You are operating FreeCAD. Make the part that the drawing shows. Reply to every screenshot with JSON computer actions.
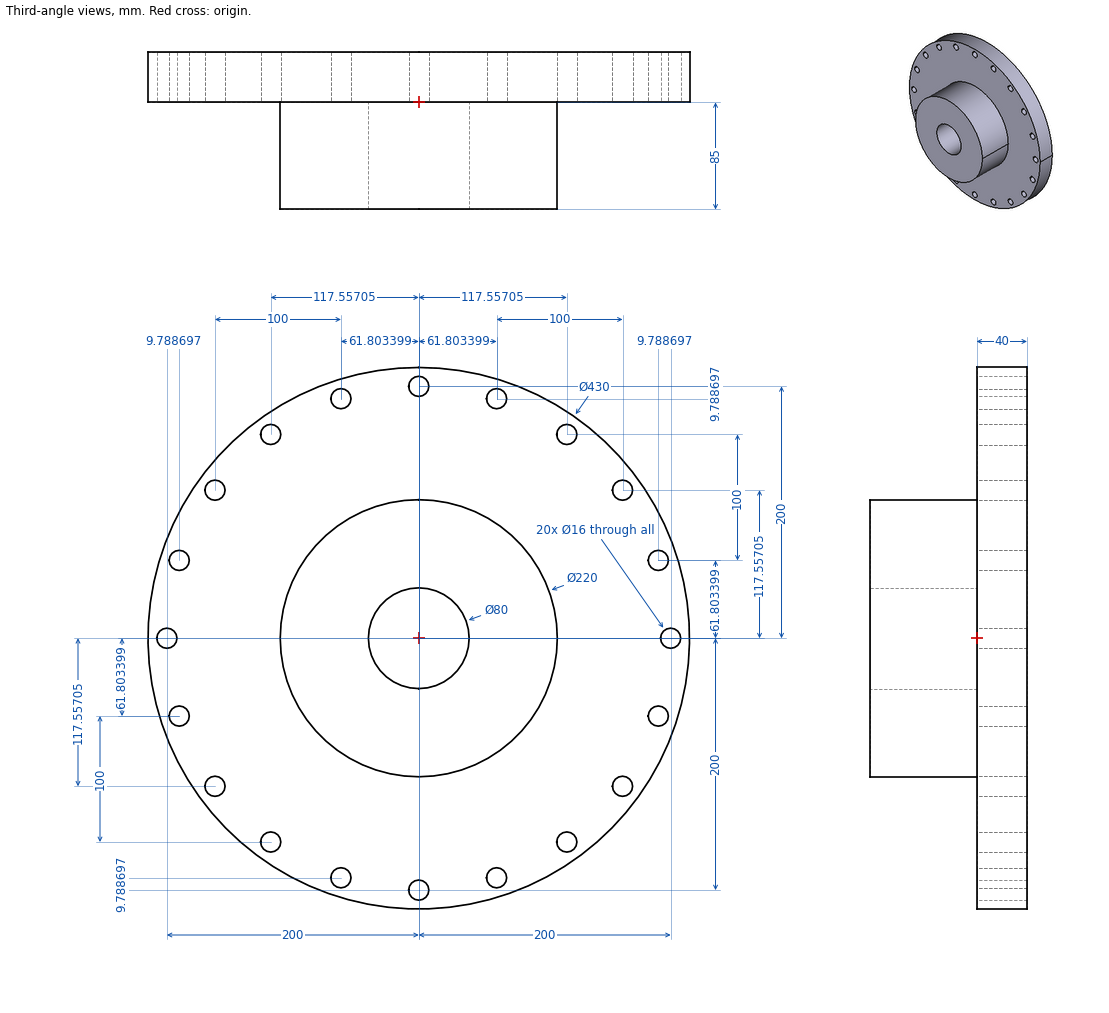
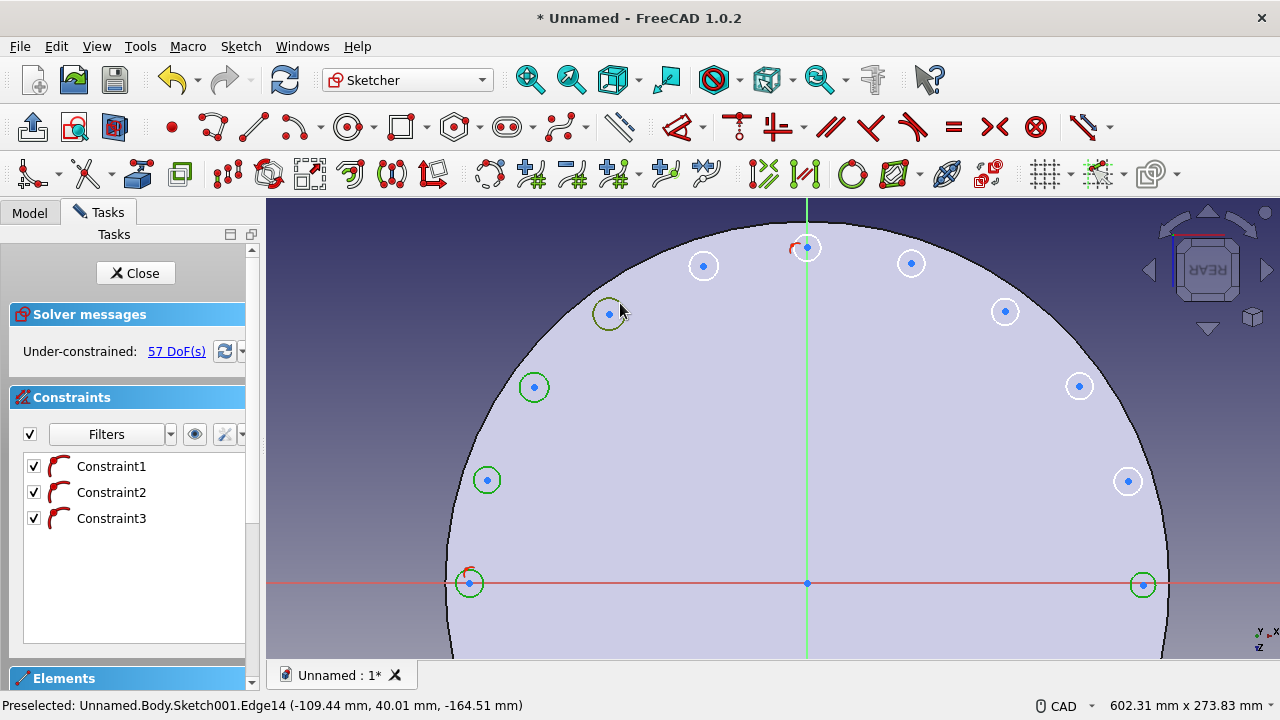
{"action": "left_click", "coordinate": [714, 256]}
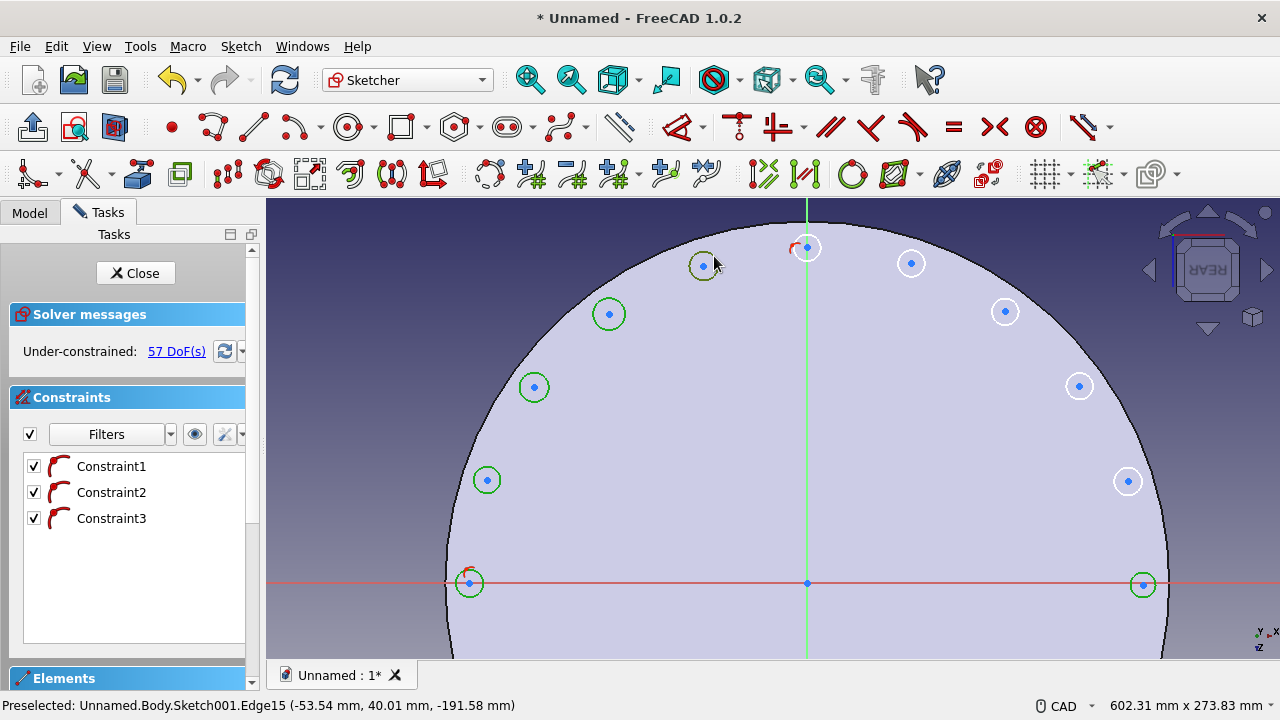
{"action": "scroll", "coordinate": [817, 238], "scroll_direction": "up", "scroll_amount": 2}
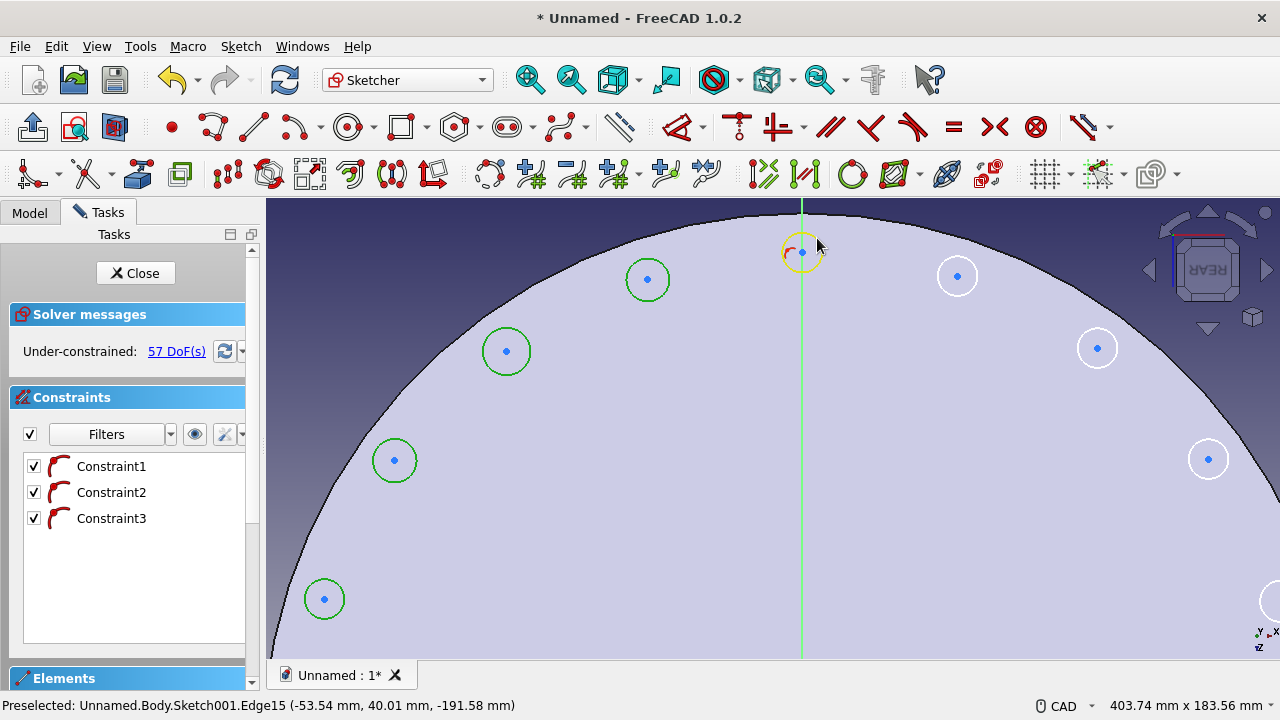
{"action": "left_click", "coordinate": [816, 239]}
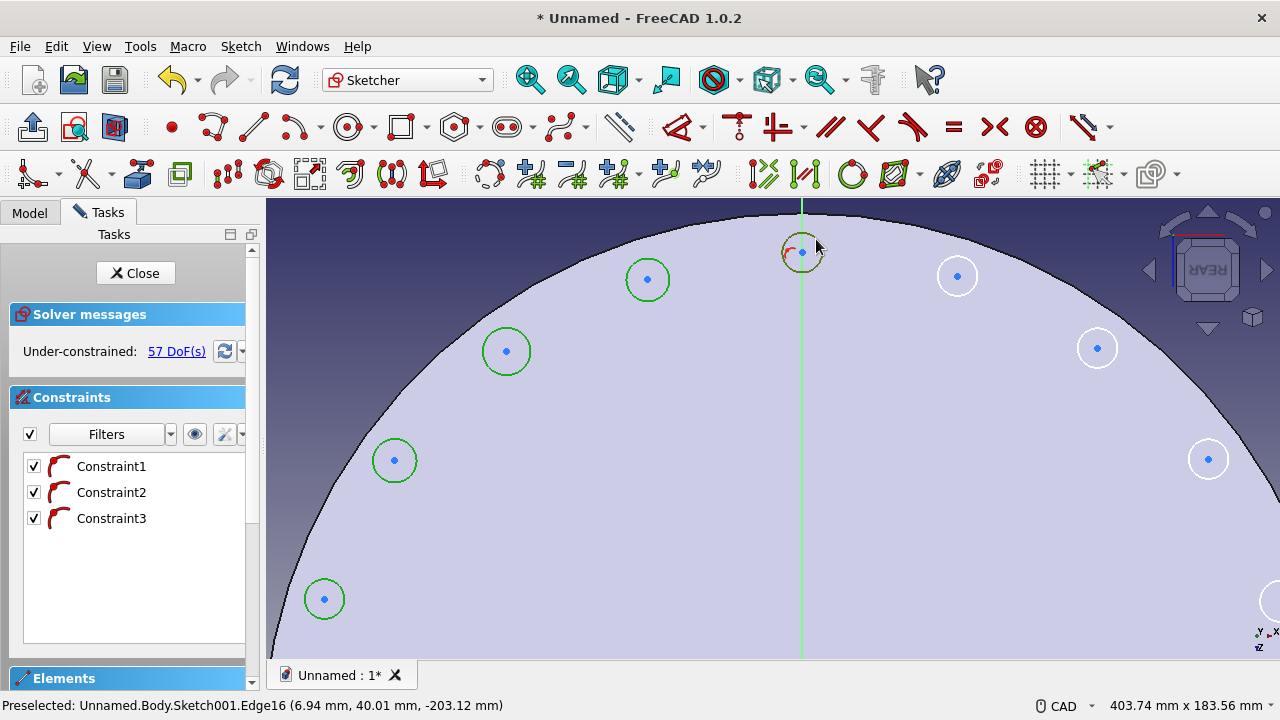
{"action": "left_click", "coordinate": [972, 262]}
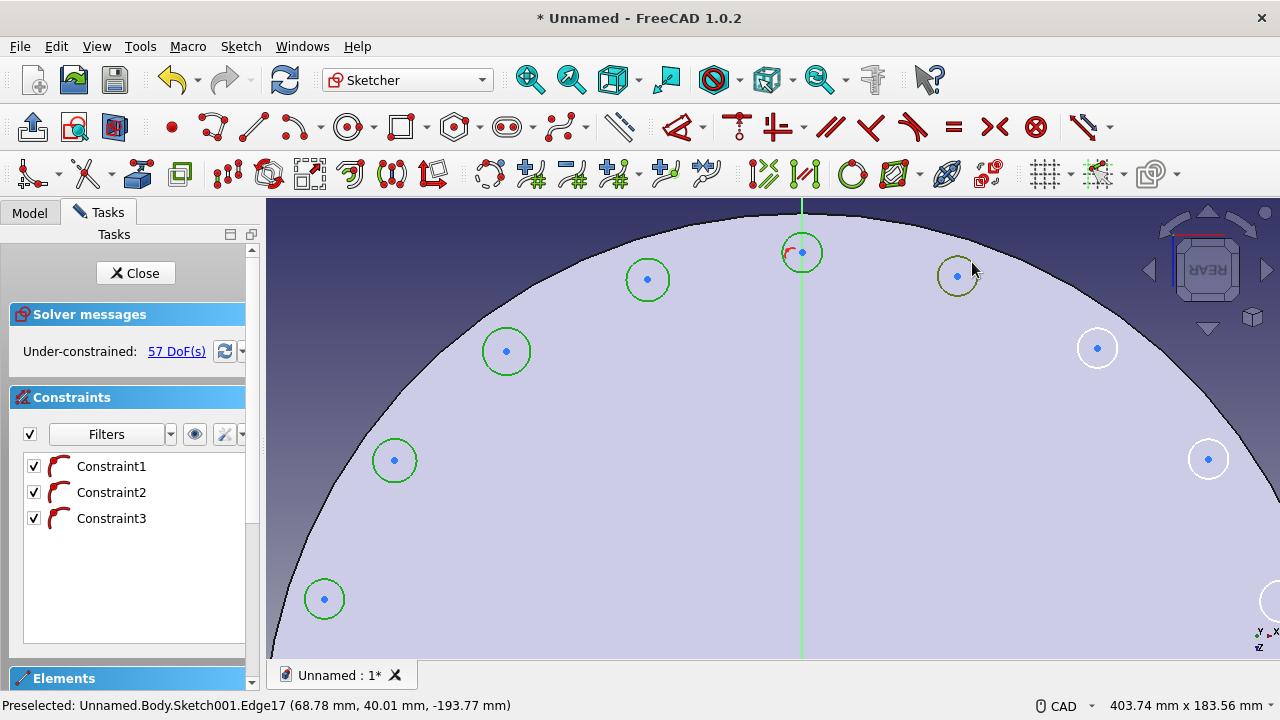
{"action": "left_click", "coordinate": [1112, 334]}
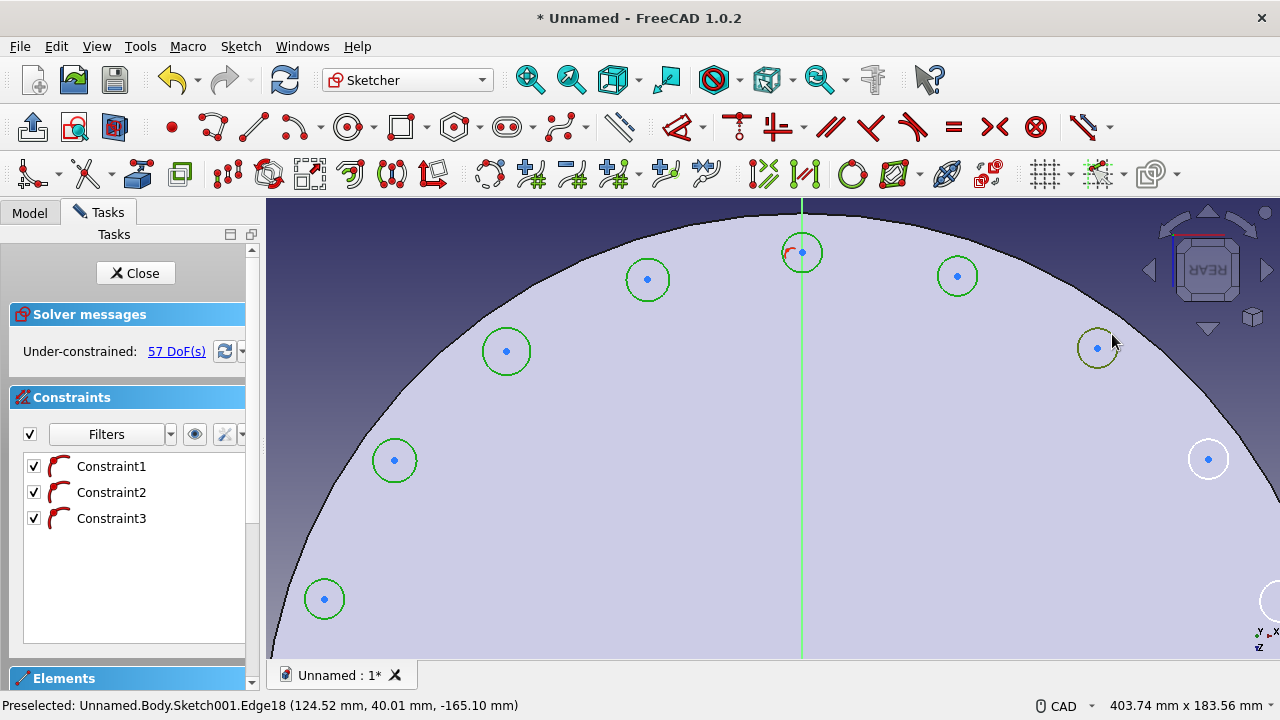
{"action": "scroll", "coordinate": [662, 289], "scroll_direction": "down", "scroll_amount": 6}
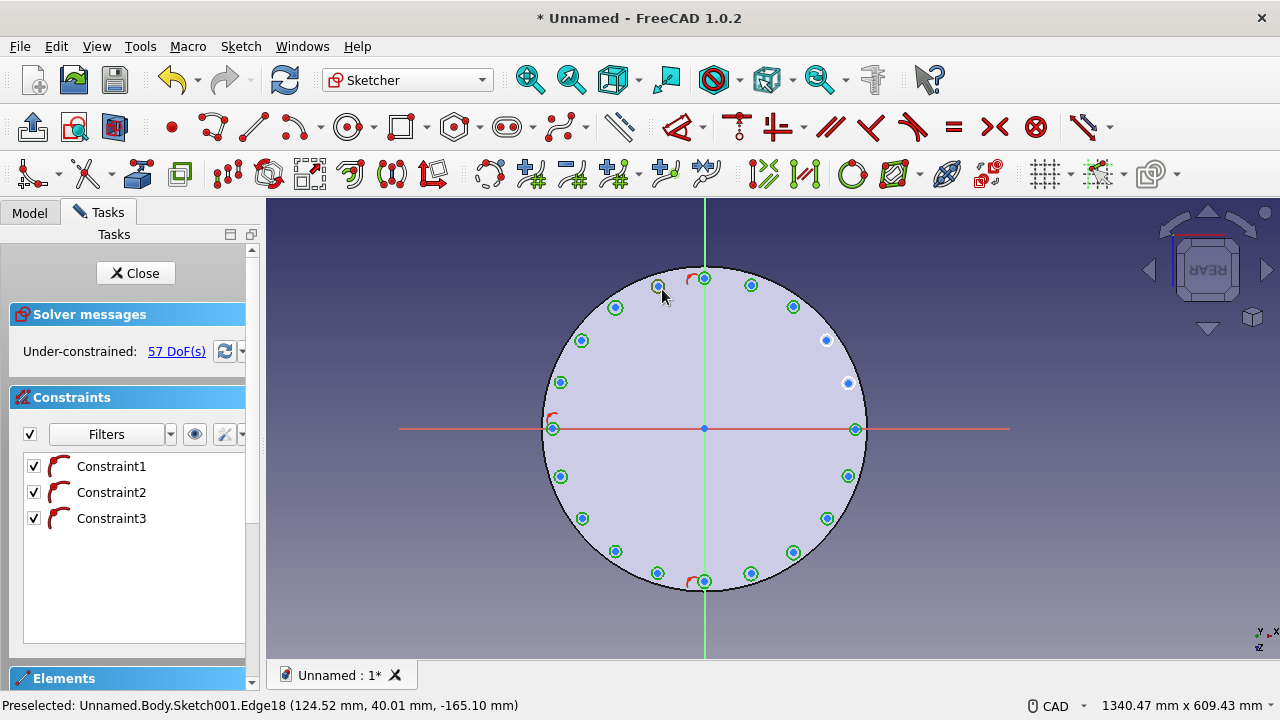
{"action": "scroll", "coordinate": [831, 336], "scroll_direction": "up", "scroll_amount": 5}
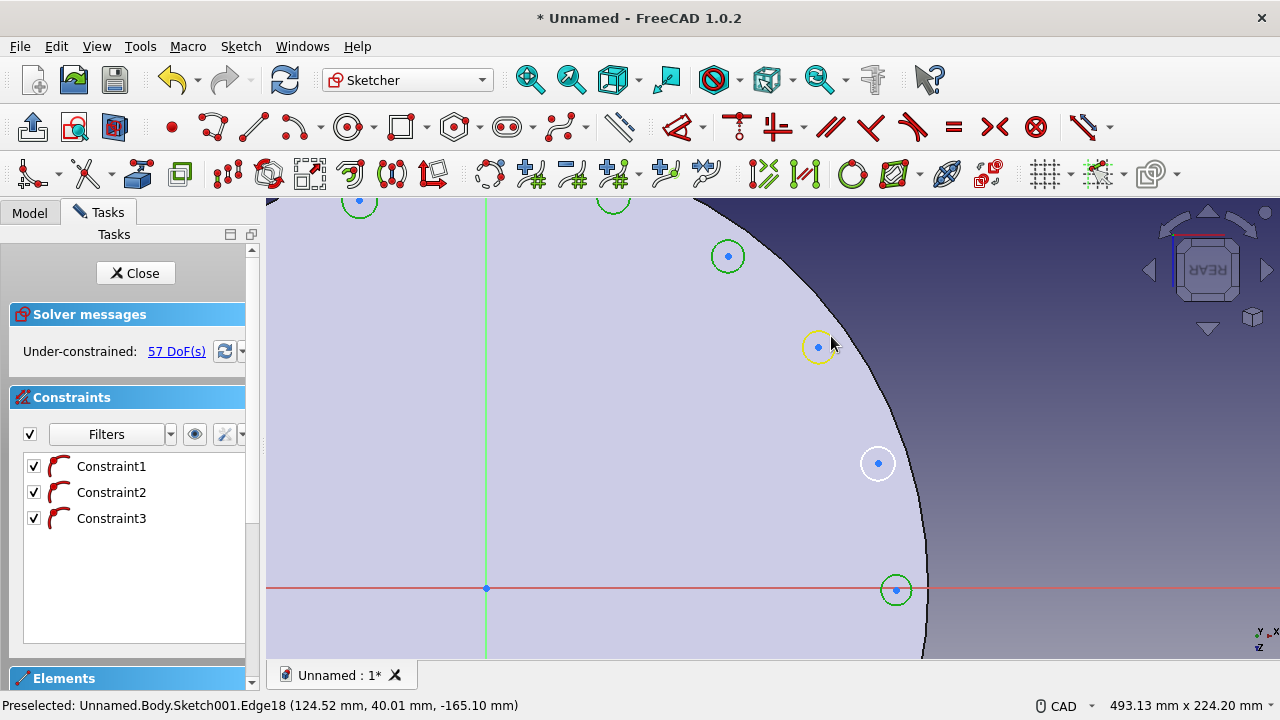
{"action": "left_click", "coordinate": [830, 336]}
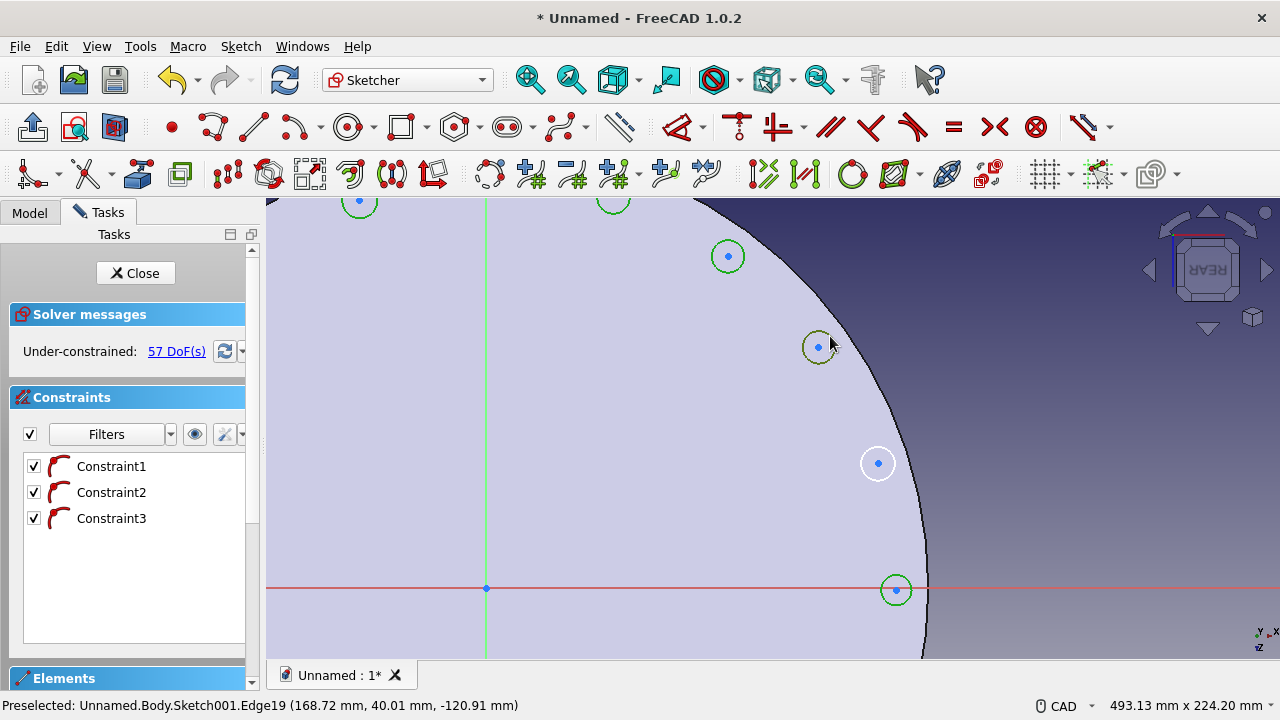
{"action": "left_click", "coordinate": [890, 452]}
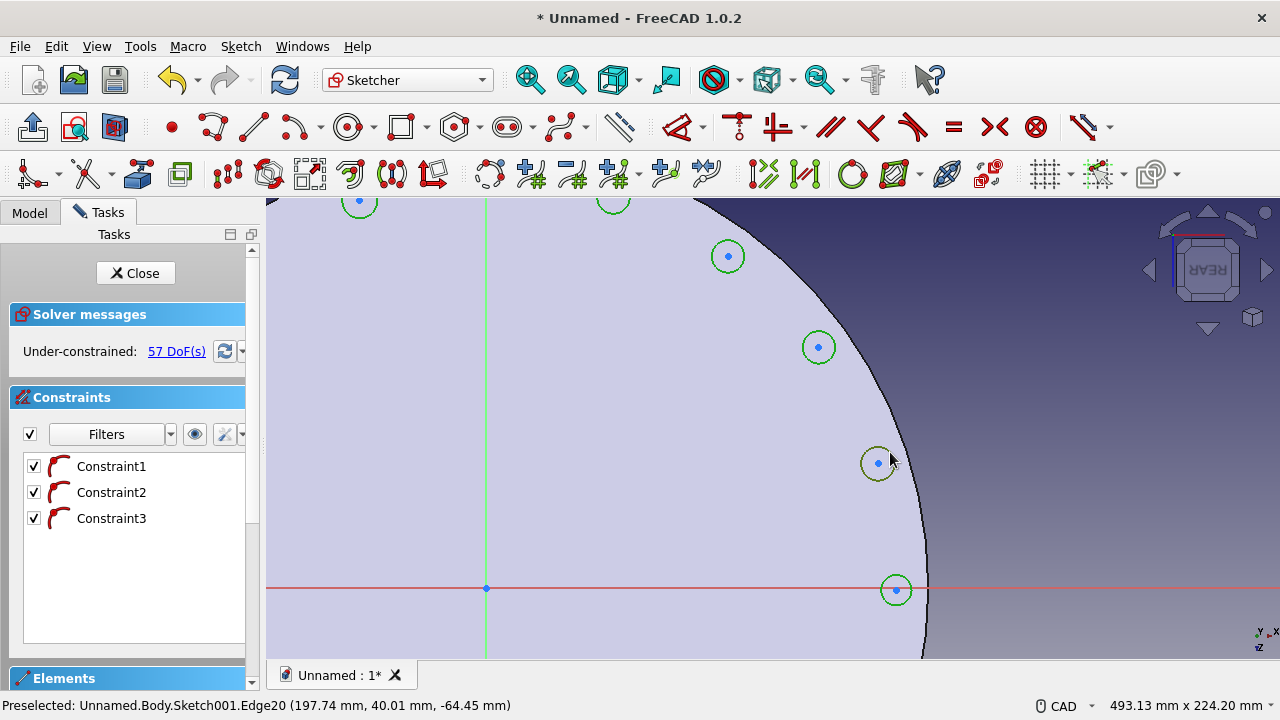
{"action": "left_click", "coordinate": [954, 128]}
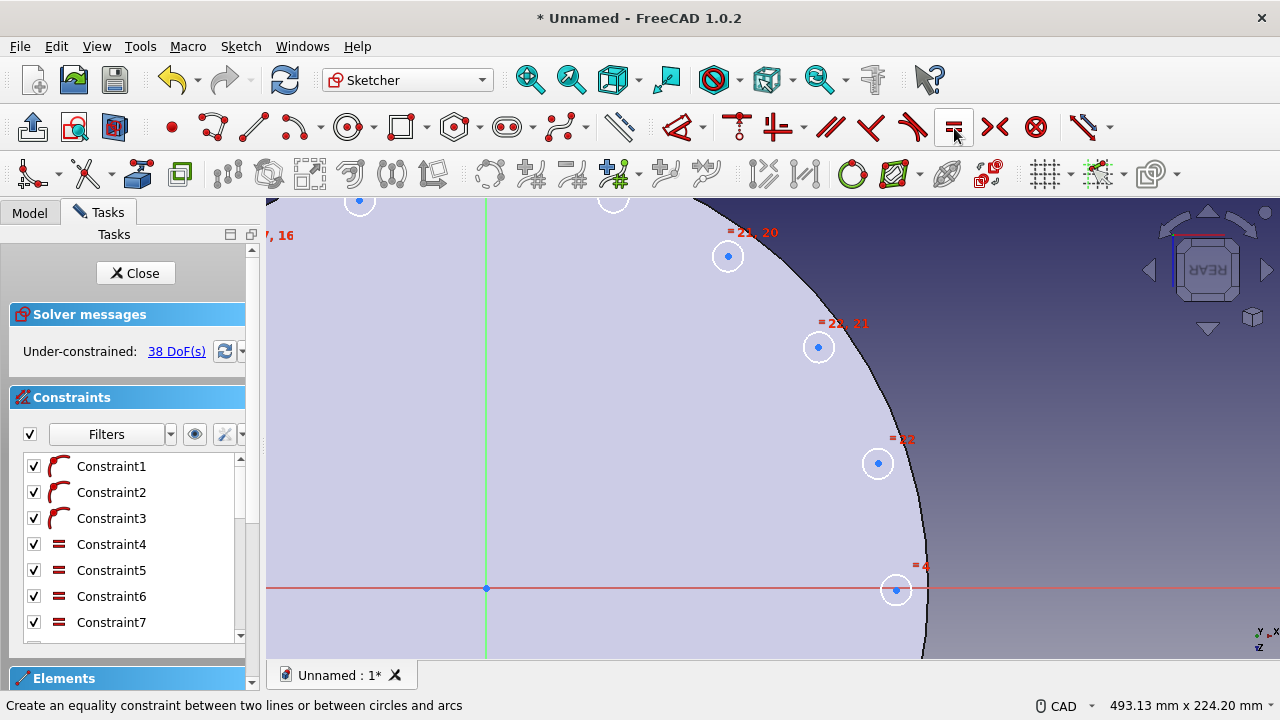
{"action": "left_click", "coordinate": [896, 590]}